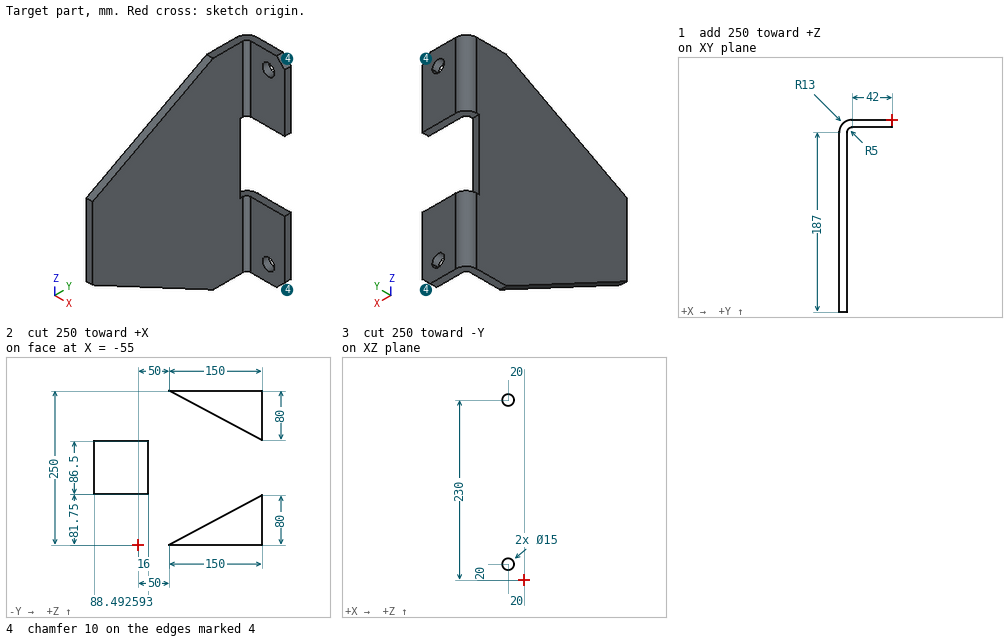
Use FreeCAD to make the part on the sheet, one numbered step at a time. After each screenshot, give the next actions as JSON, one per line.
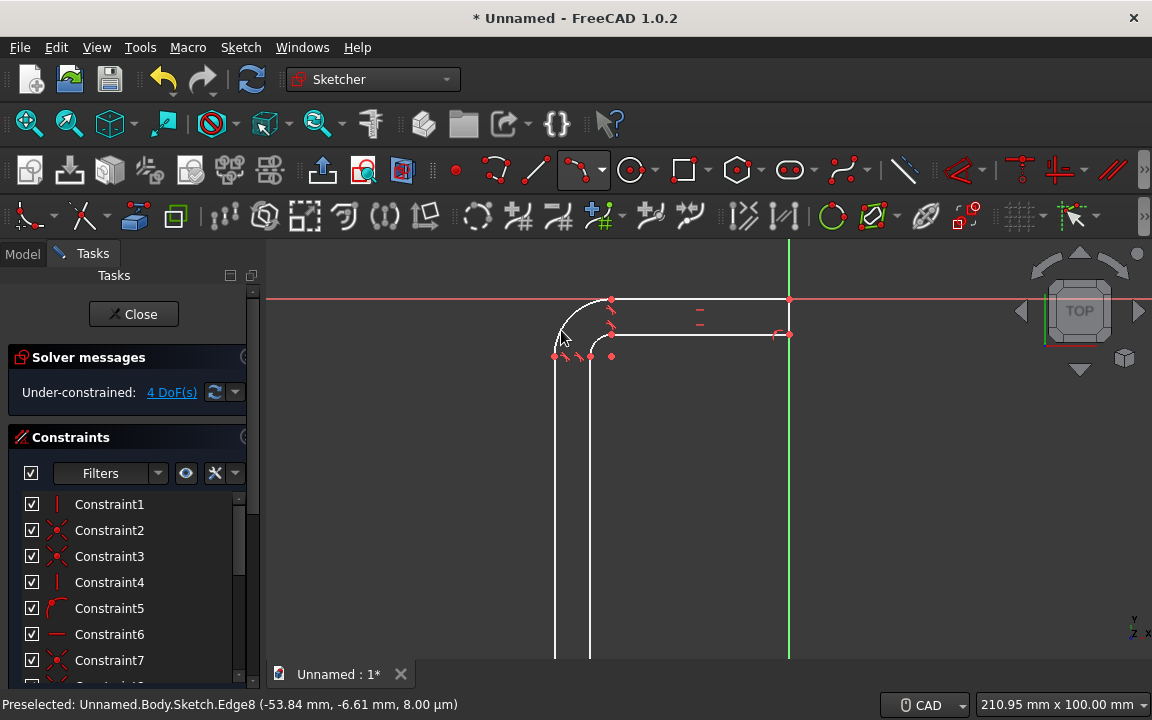
{"action": "scroll", "coordinate": [602, 337], "scroll_direction": "up", "scroll_amount": 4}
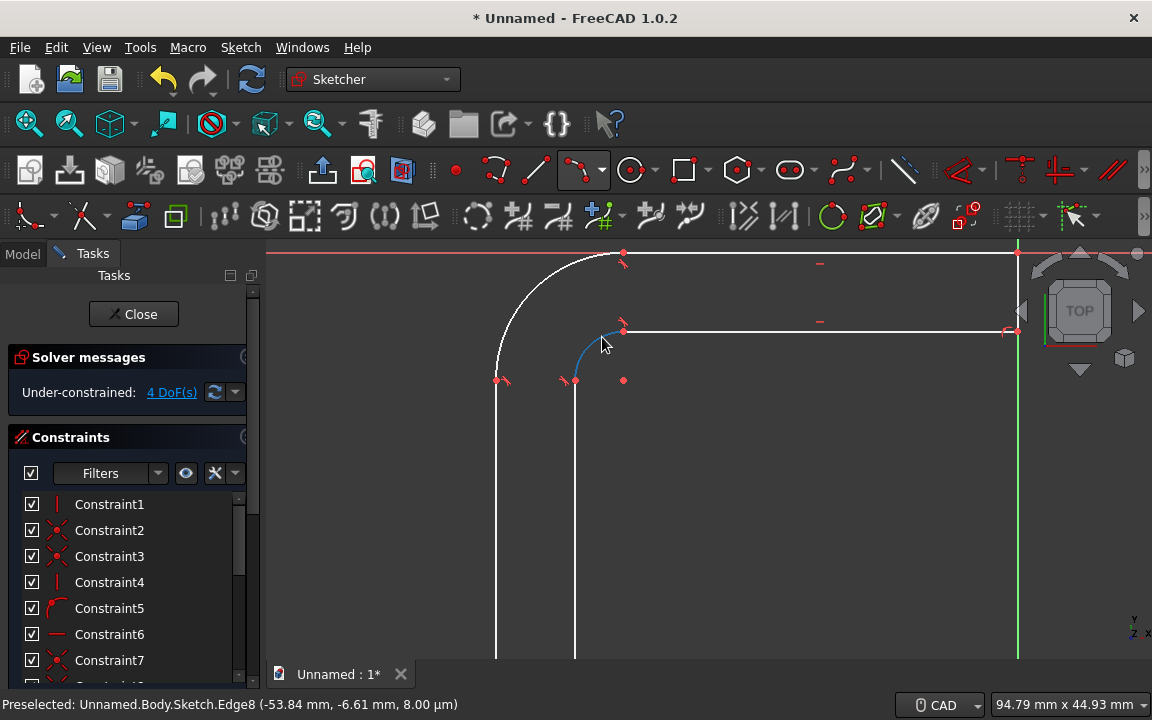
{"action": "left_click", "coordinate": [601, 337]}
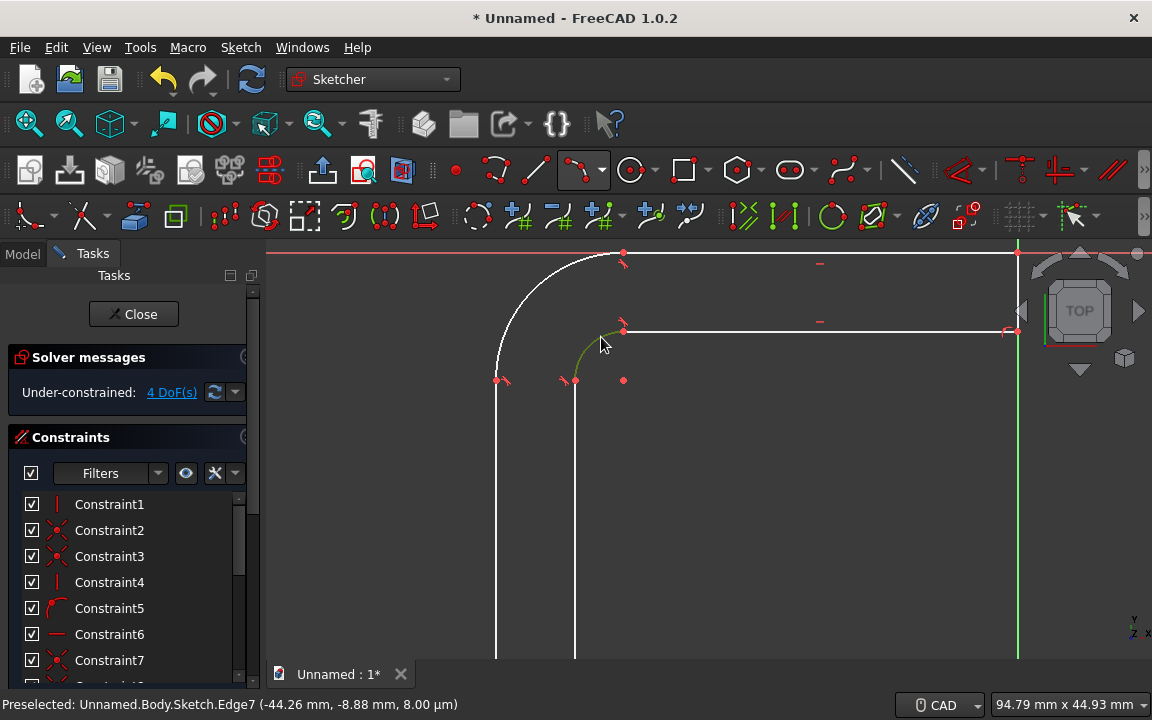
{"action": "left_click", "coordinate": [984, 170]}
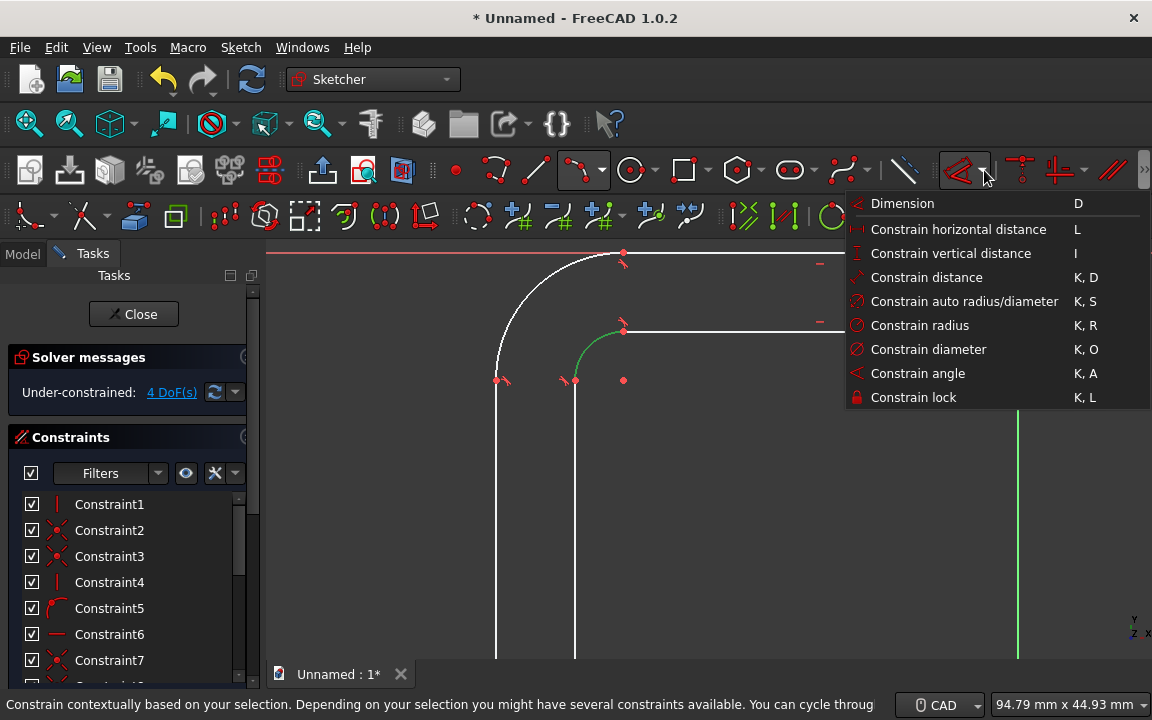
{"action": "left_click", "coordinate": [998, 325]}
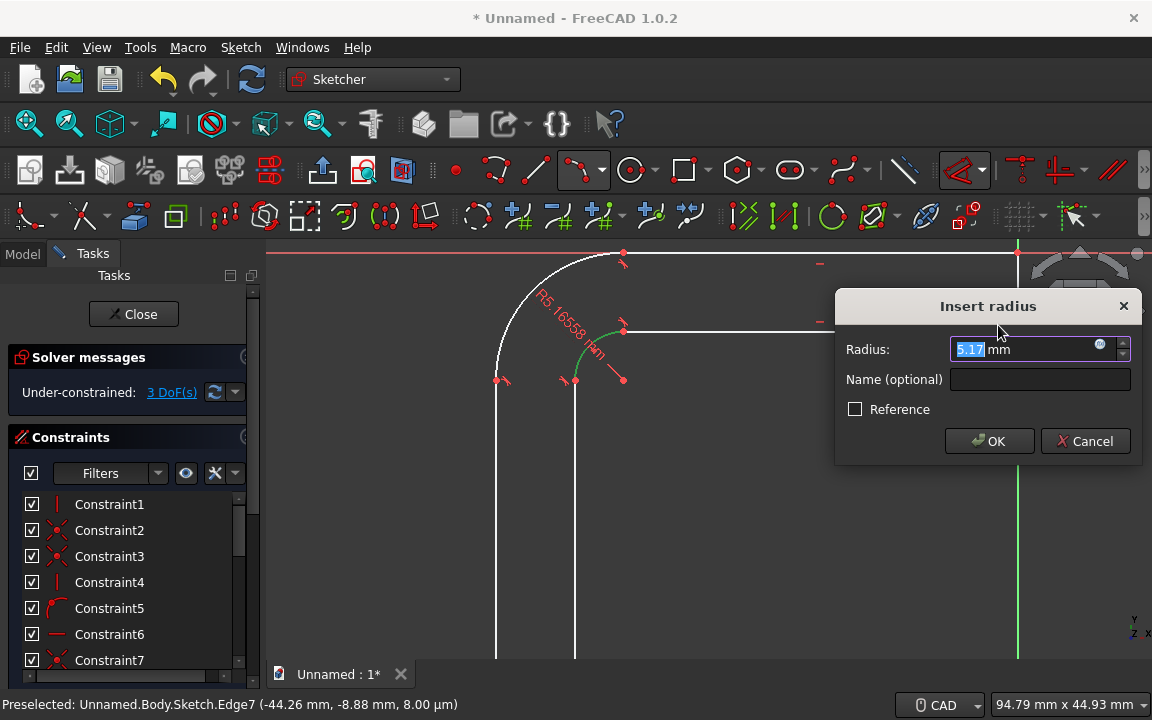
{"action": "type", "text": "5"}
{"action": "key", "text": "Return"}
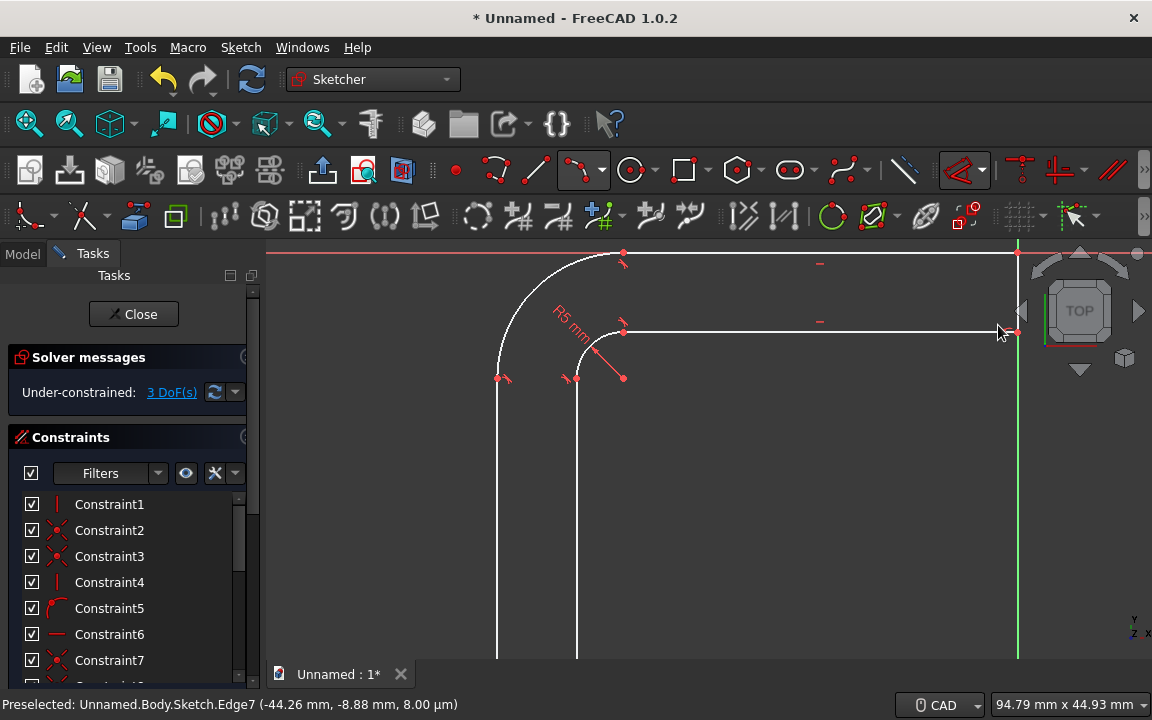
{"action": "scroll", "coordinate": [622, 333], "scroll_direction": "down", "scroll_amount": 10}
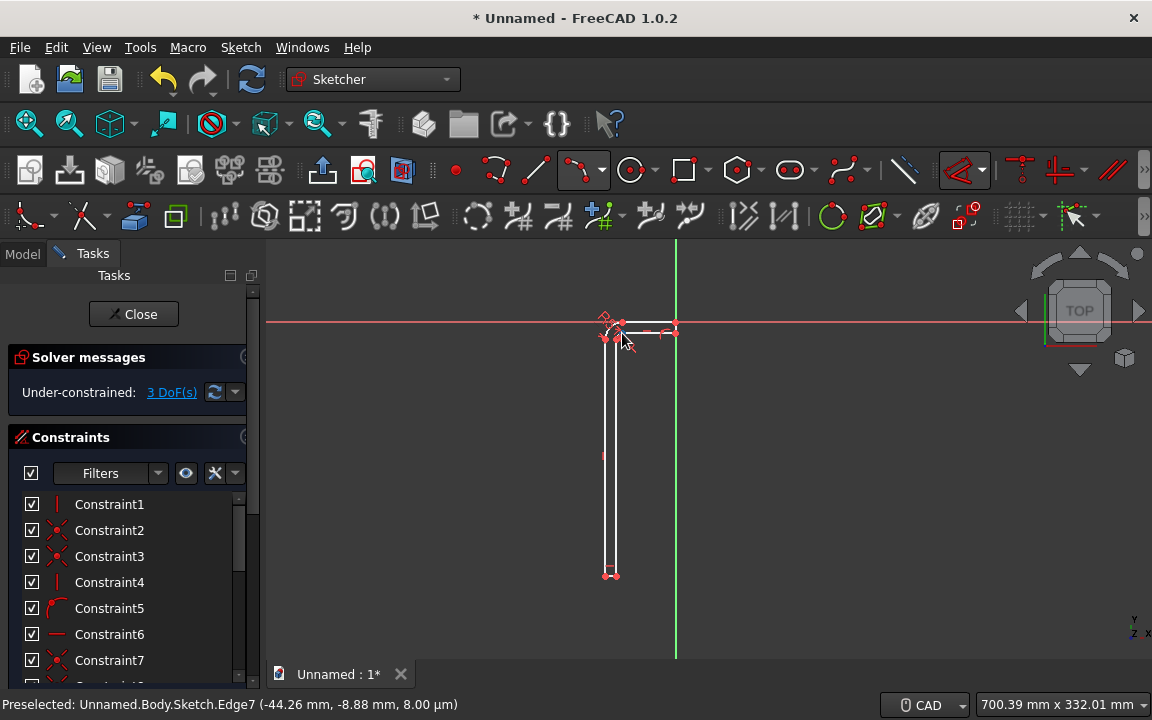
{"action": "scroll", "coordinate": [607, 332], "scroll_direction": "up", "scroll_amount": 5}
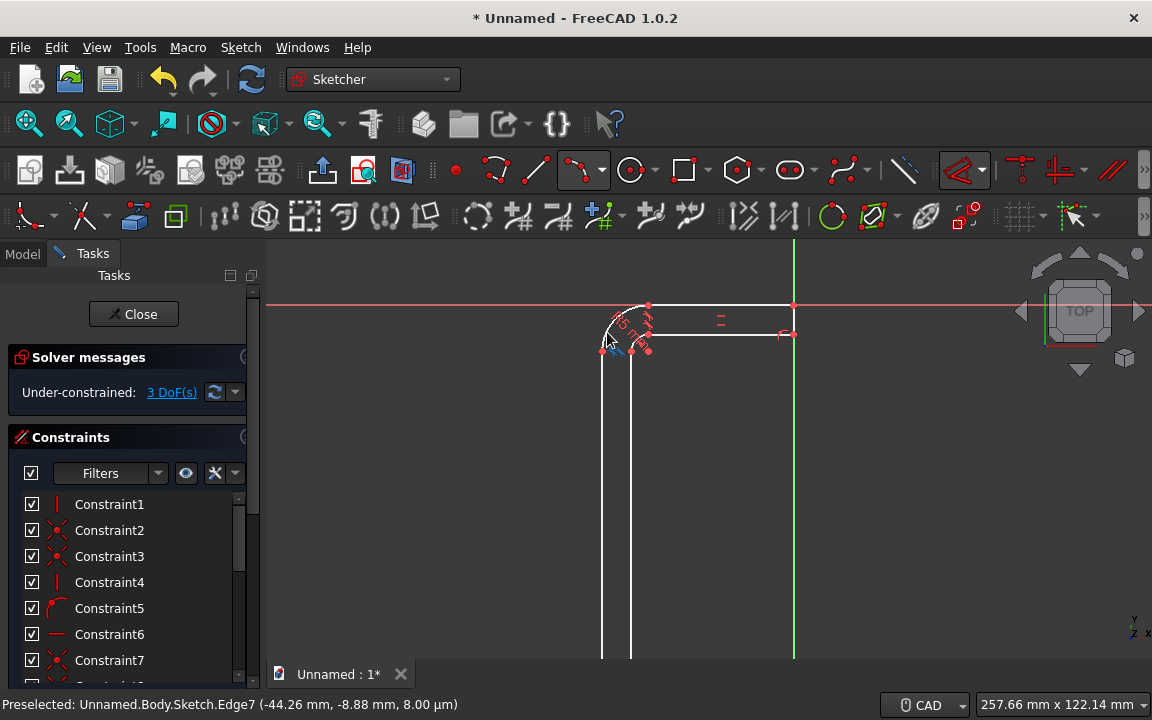
{"action": "left_click", "coordinate": [607, 331]}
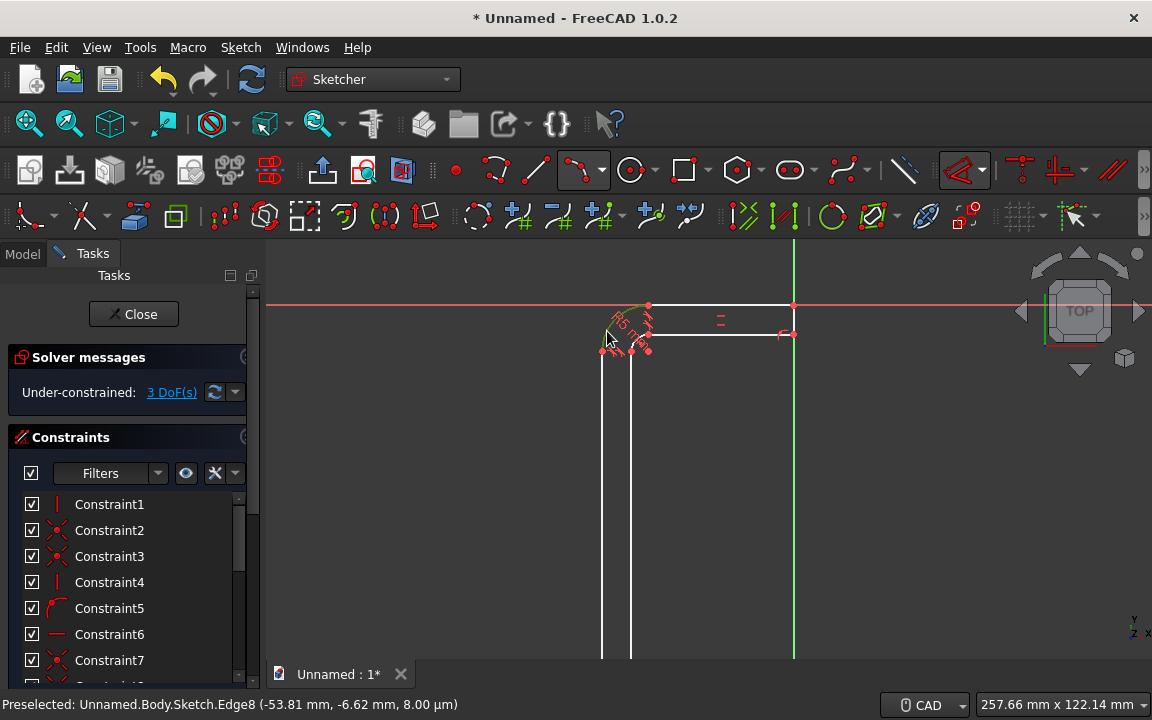
{"action": "left_click", "coordinate": [984, 170]}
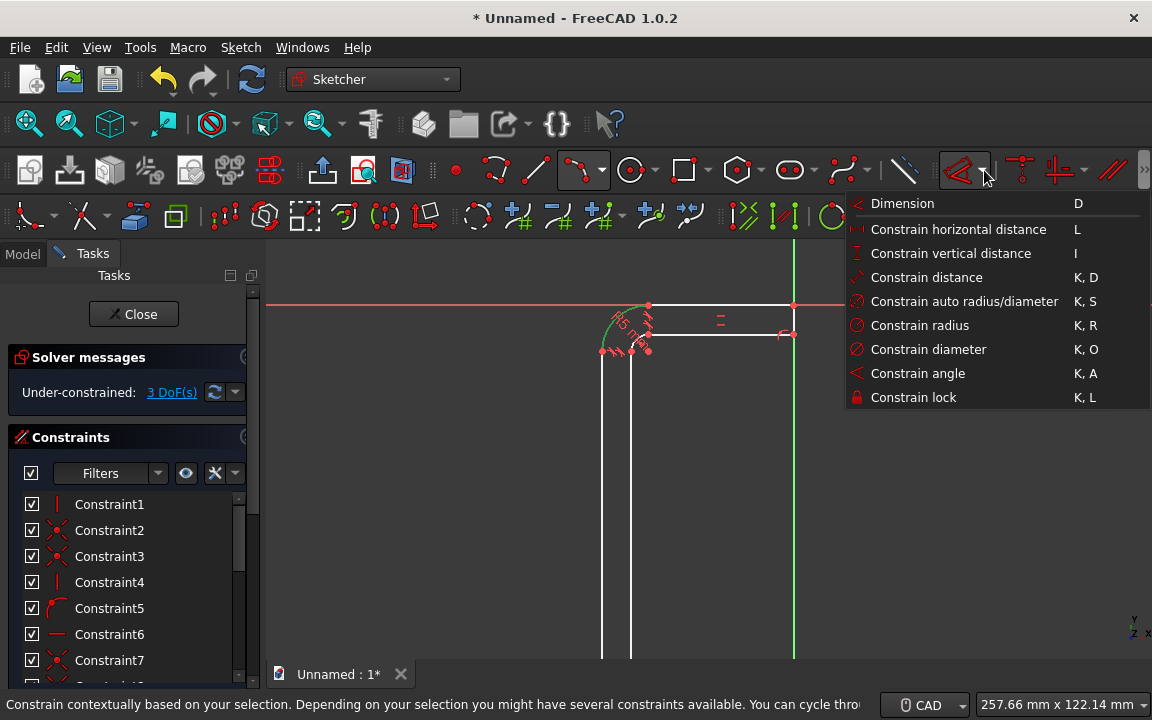
{"action": "left_click", "coordinate": [998, 325]}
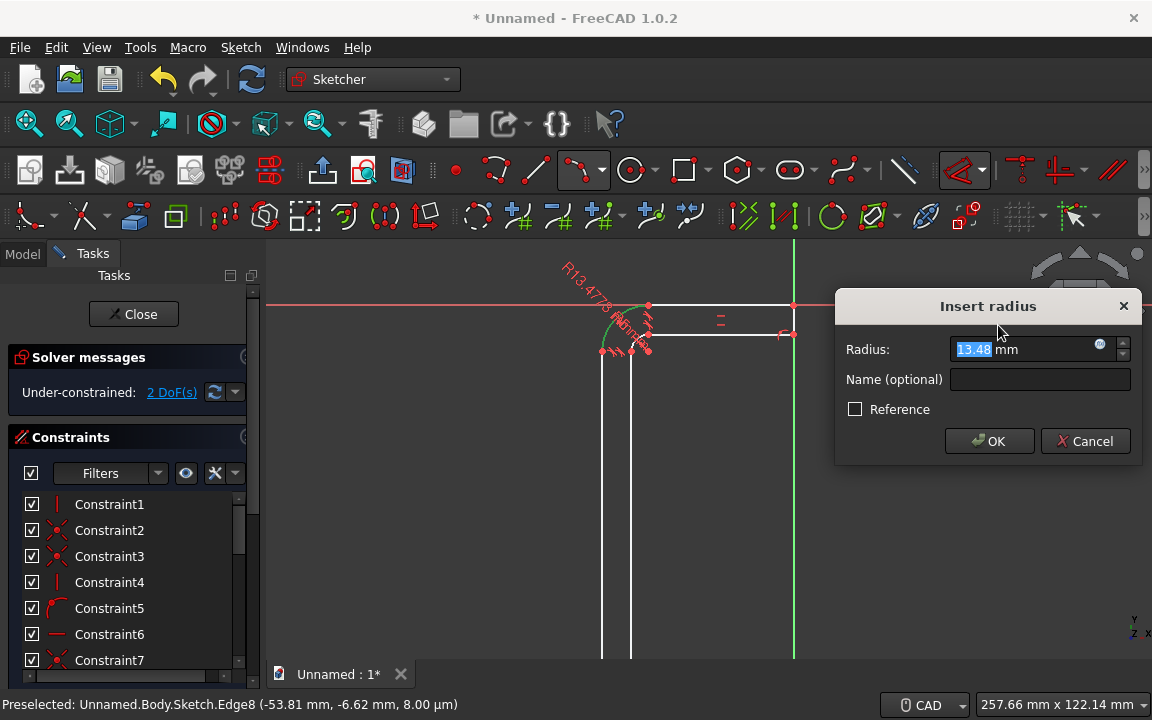
{"action": "type", "text": "13"}
{"action": "key", "text": "Return"}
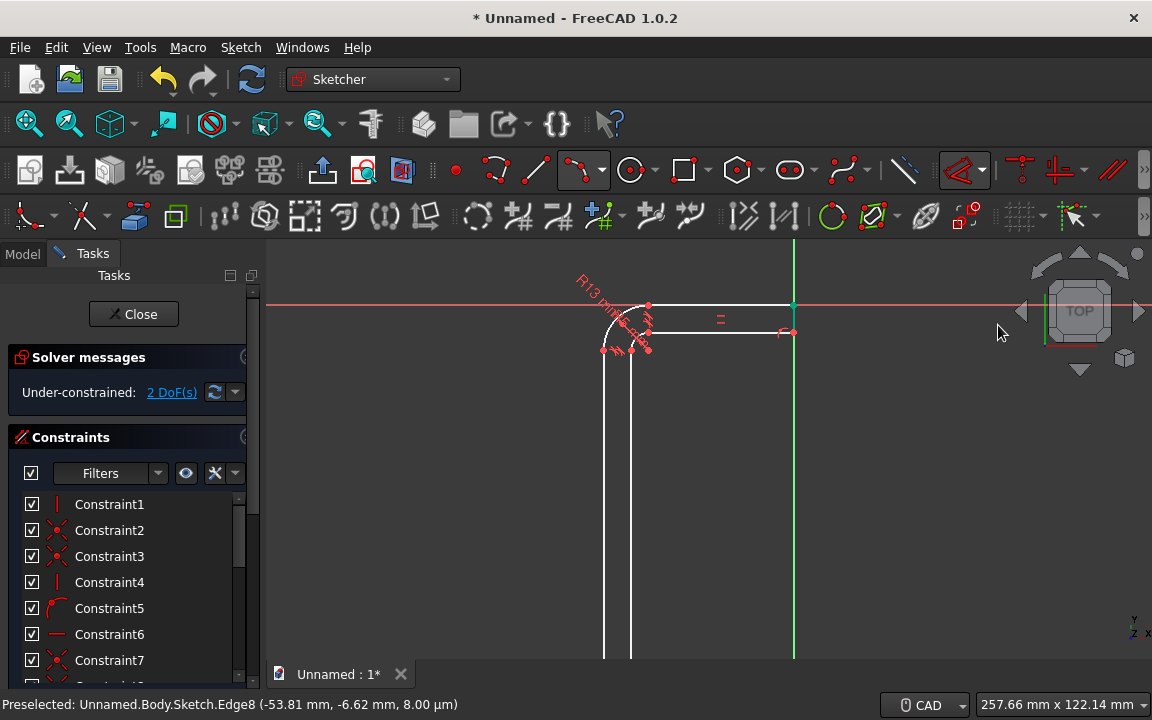
{"action": "left_click", "coordinate": [692, 333]}